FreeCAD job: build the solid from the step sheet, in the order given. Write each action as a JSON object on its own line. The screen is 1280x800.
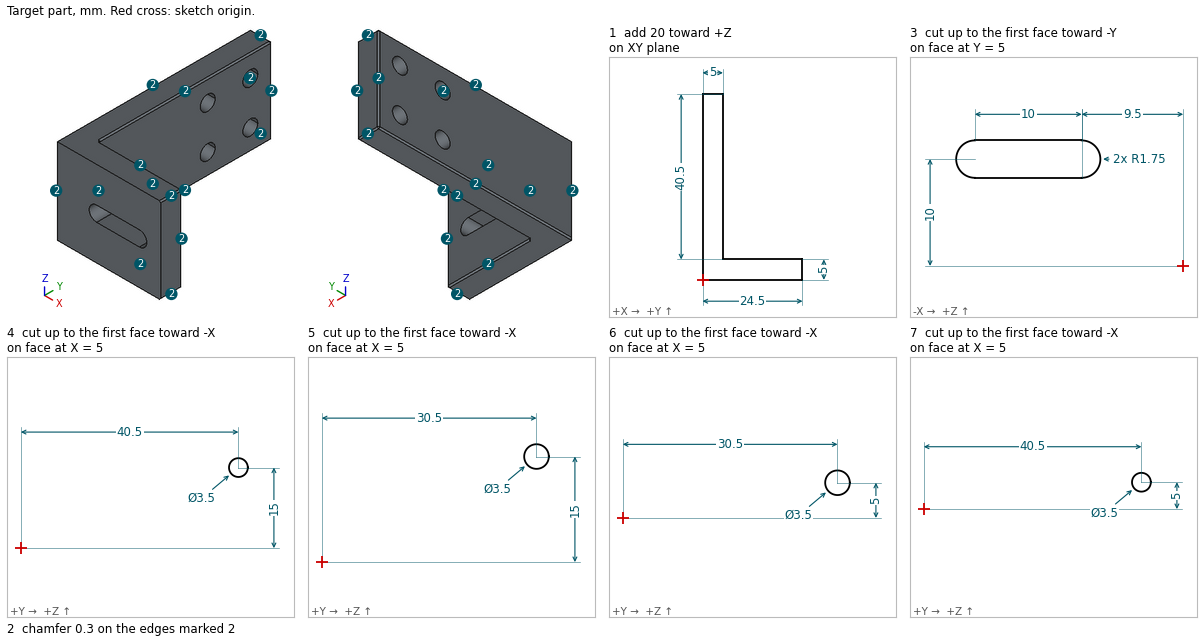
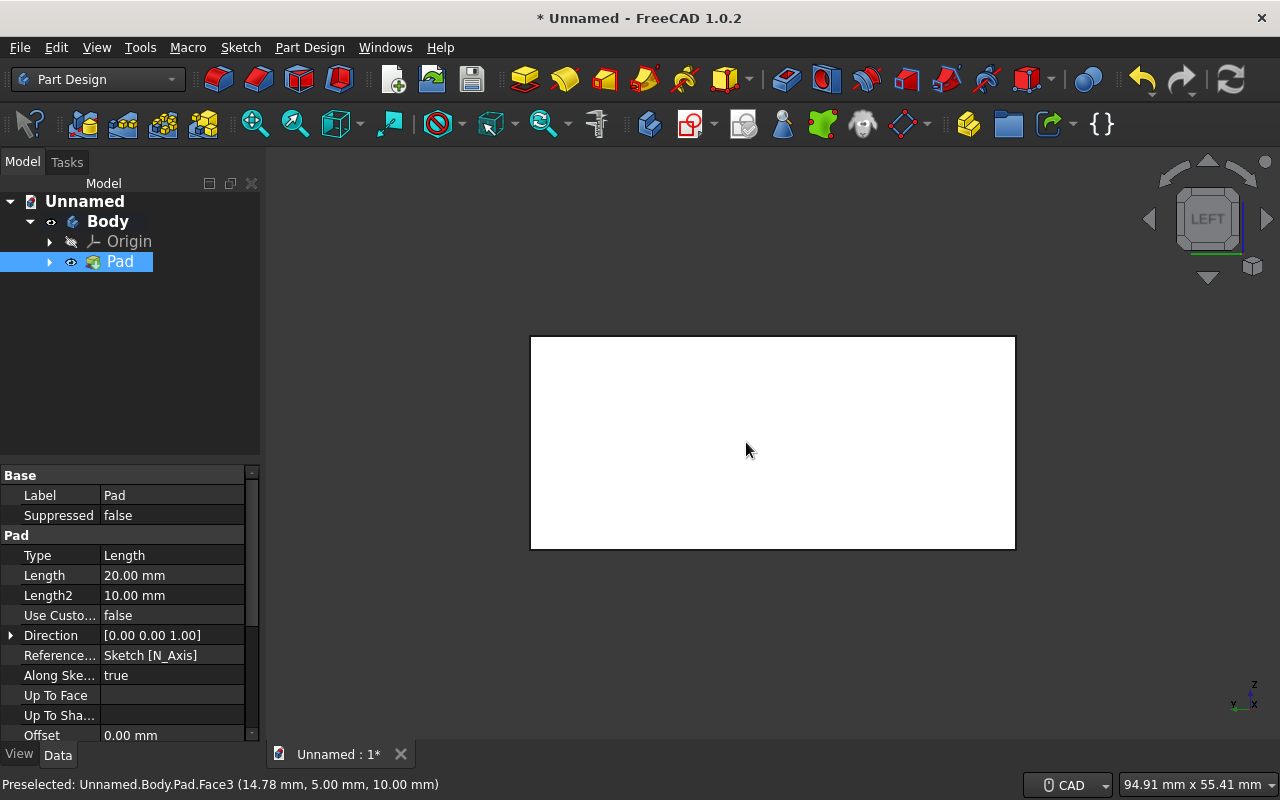
{"action": "left_click", "coordinate": [704, 442], "text": "ctrl"}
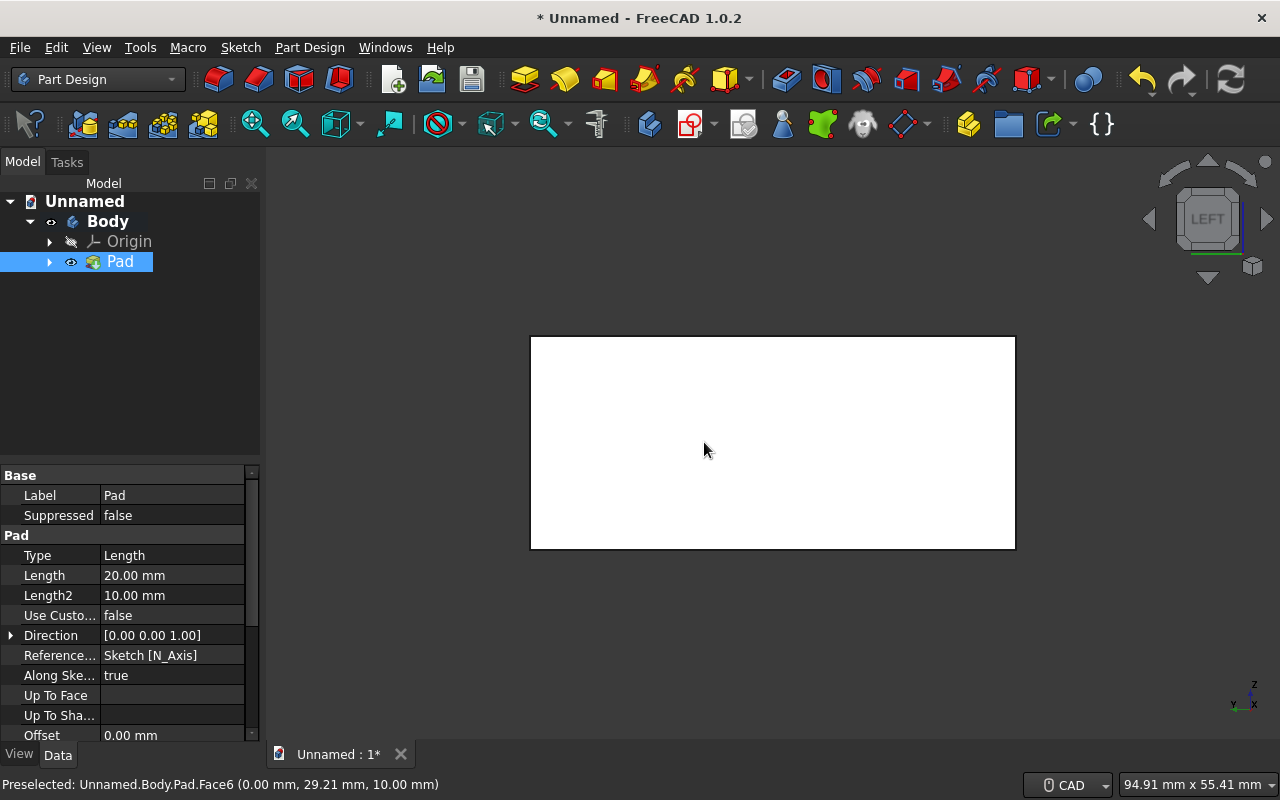
{"action": "left_click", "coordinate": [260, 80]}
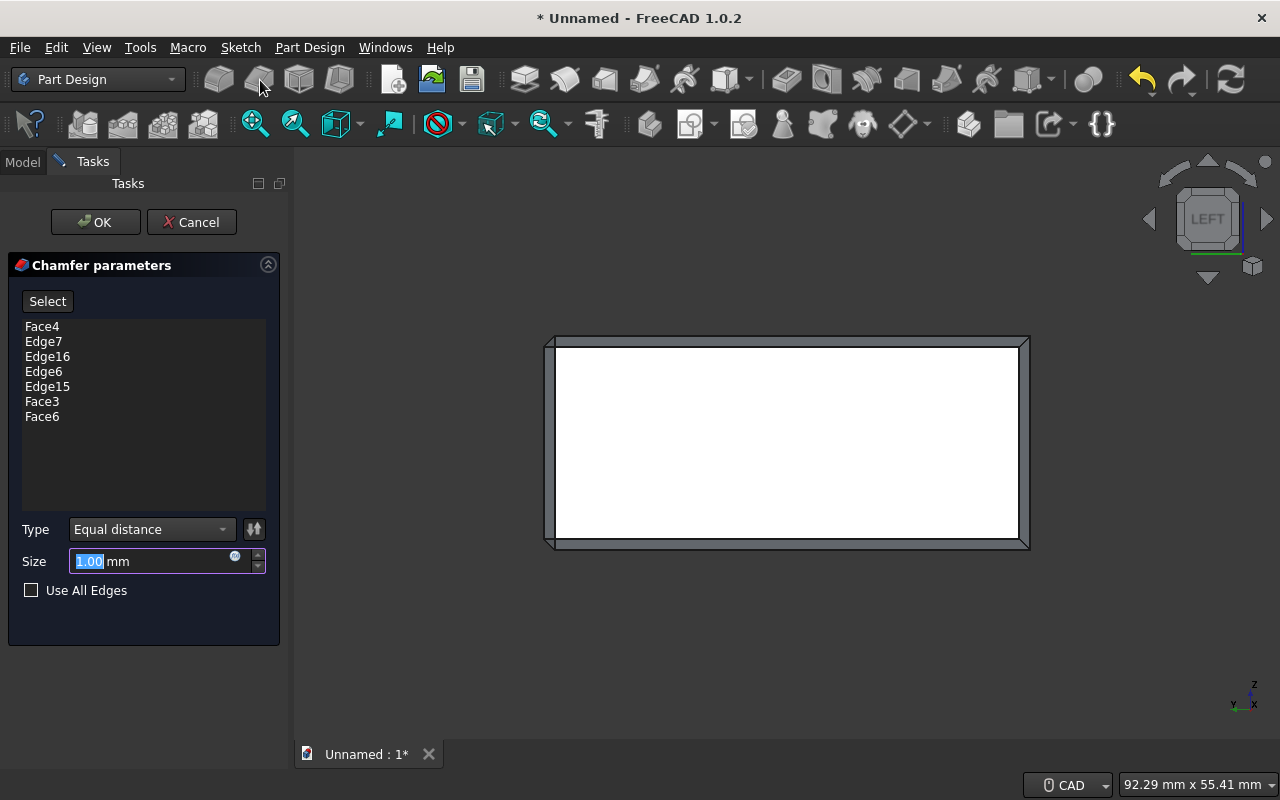
{"action": "type", "text": "0.3"}
{"action": "key", "text": "Tab"}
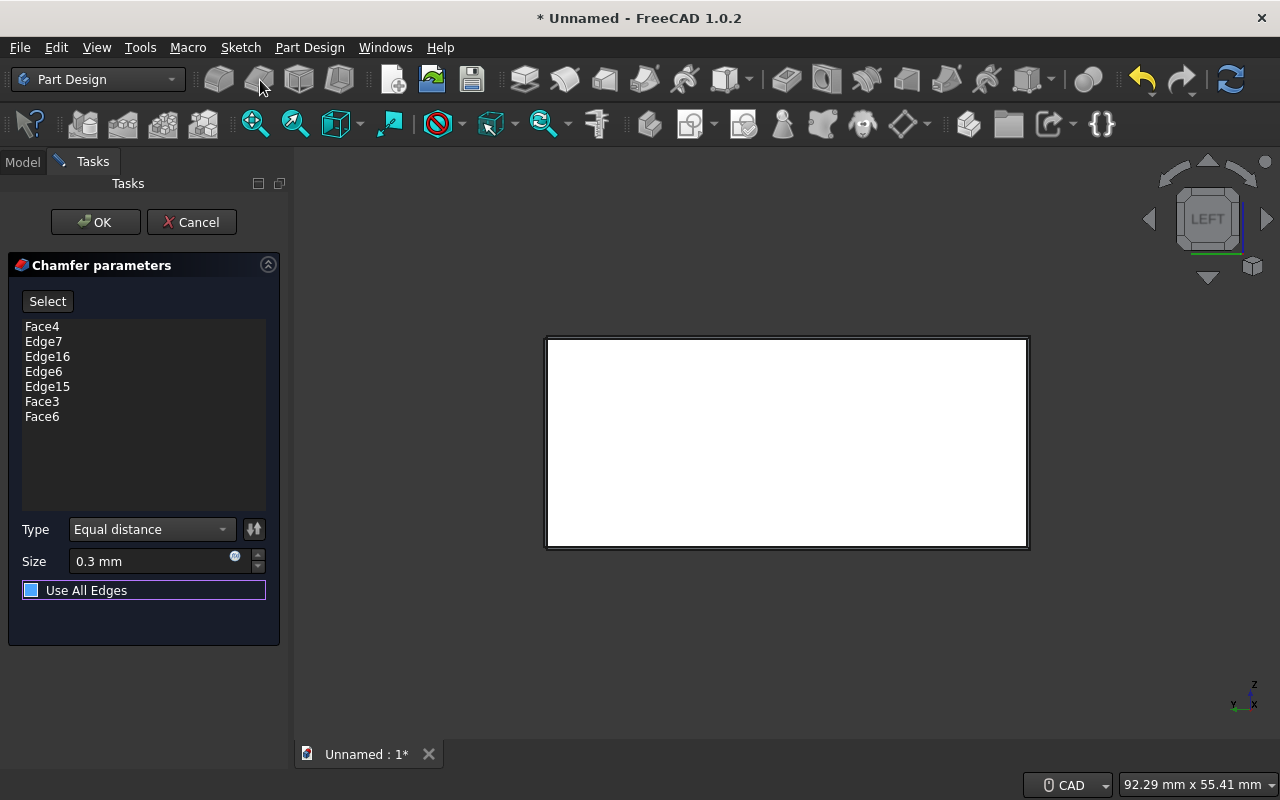
{"action": "left_click", "coordinate": [96, 222]}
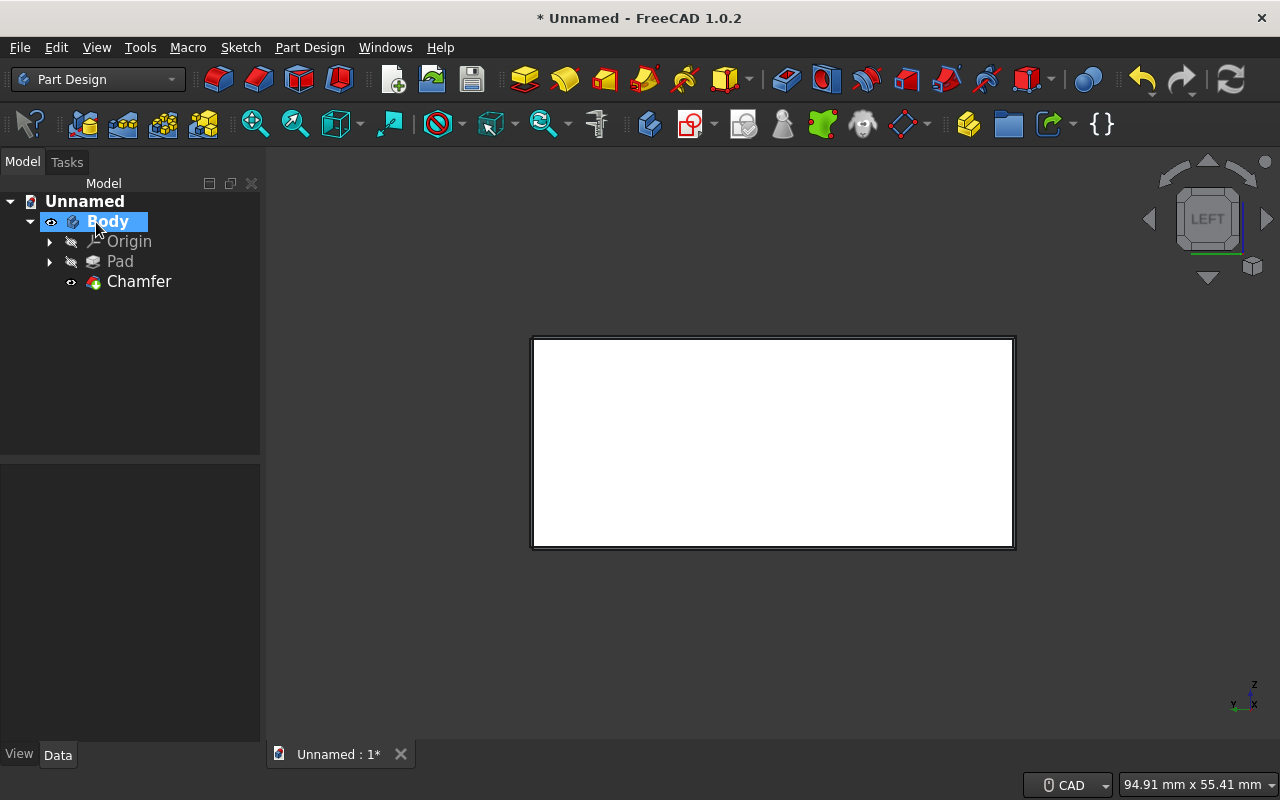
{"action": "key", "text": "4"}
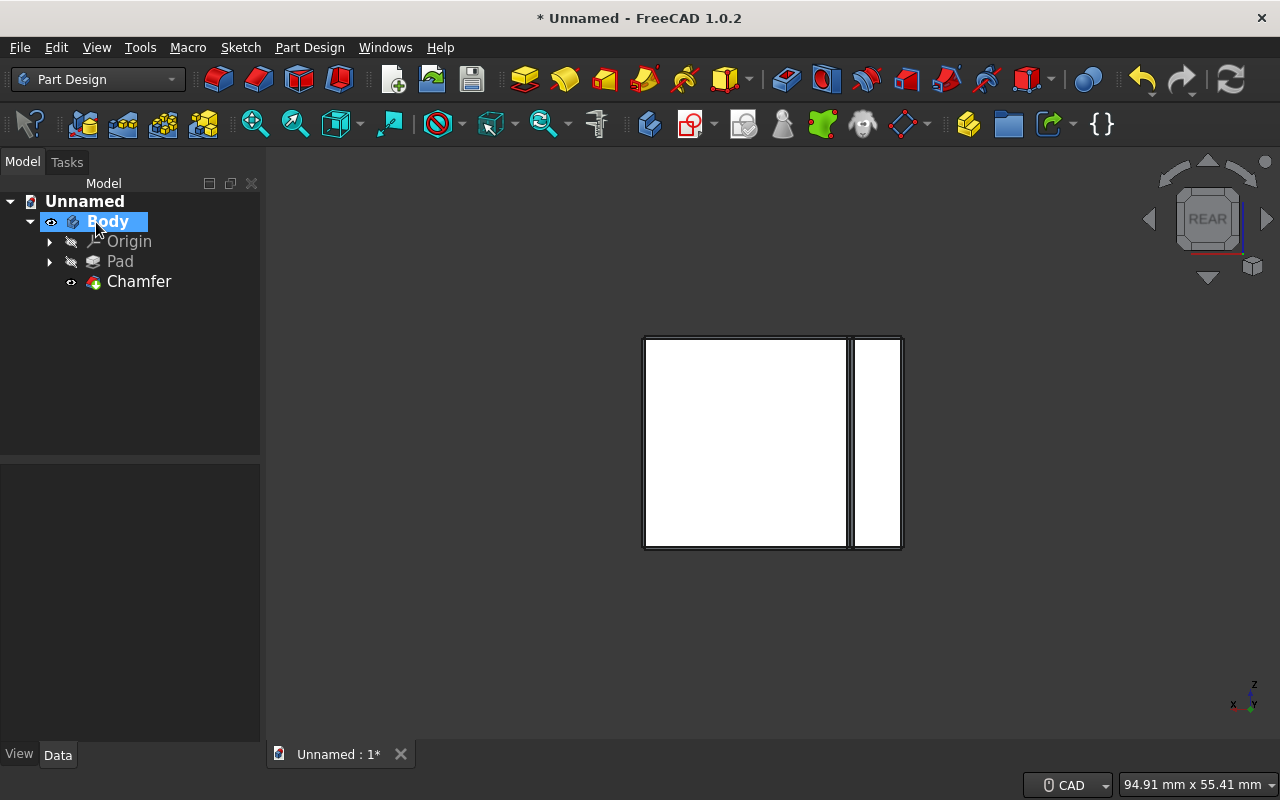
{"action": "left_click", "coordinate": [256, 124]}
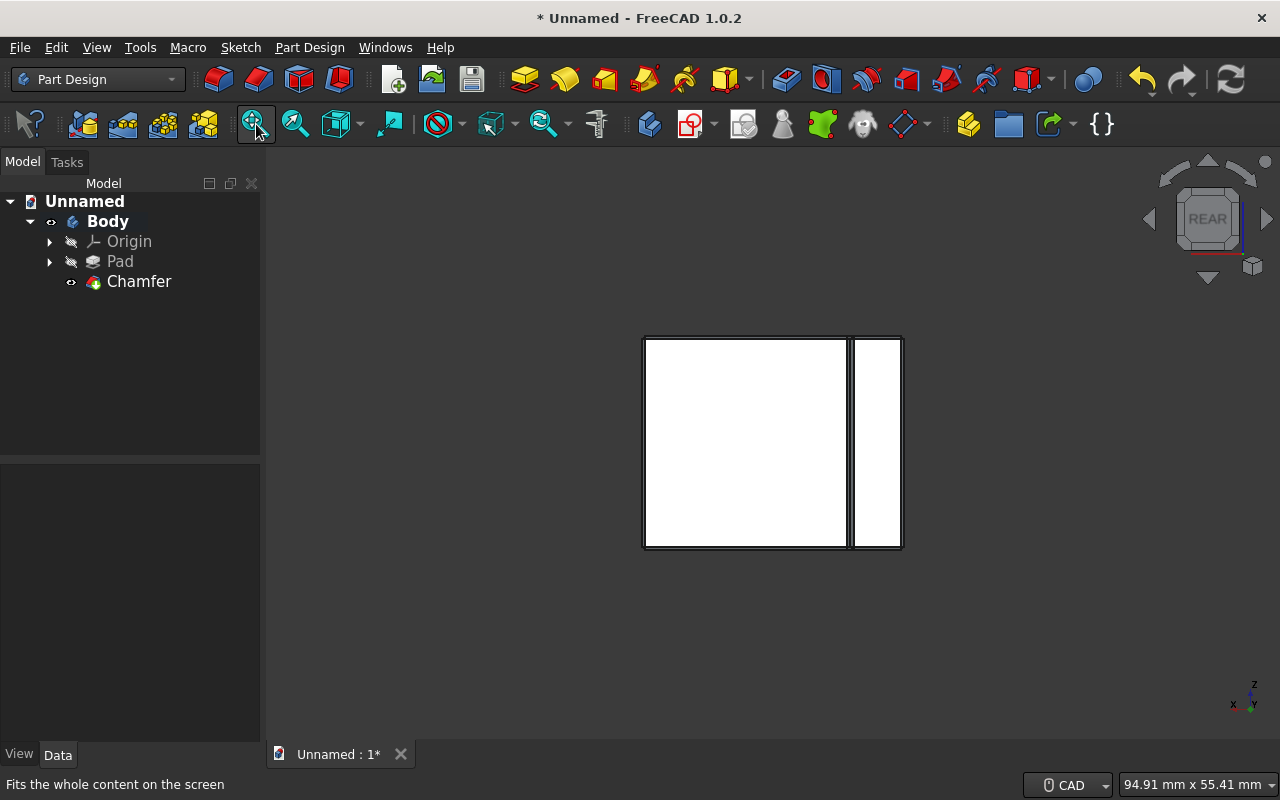
{"action": "left_click", "coordinate": [746, 442]}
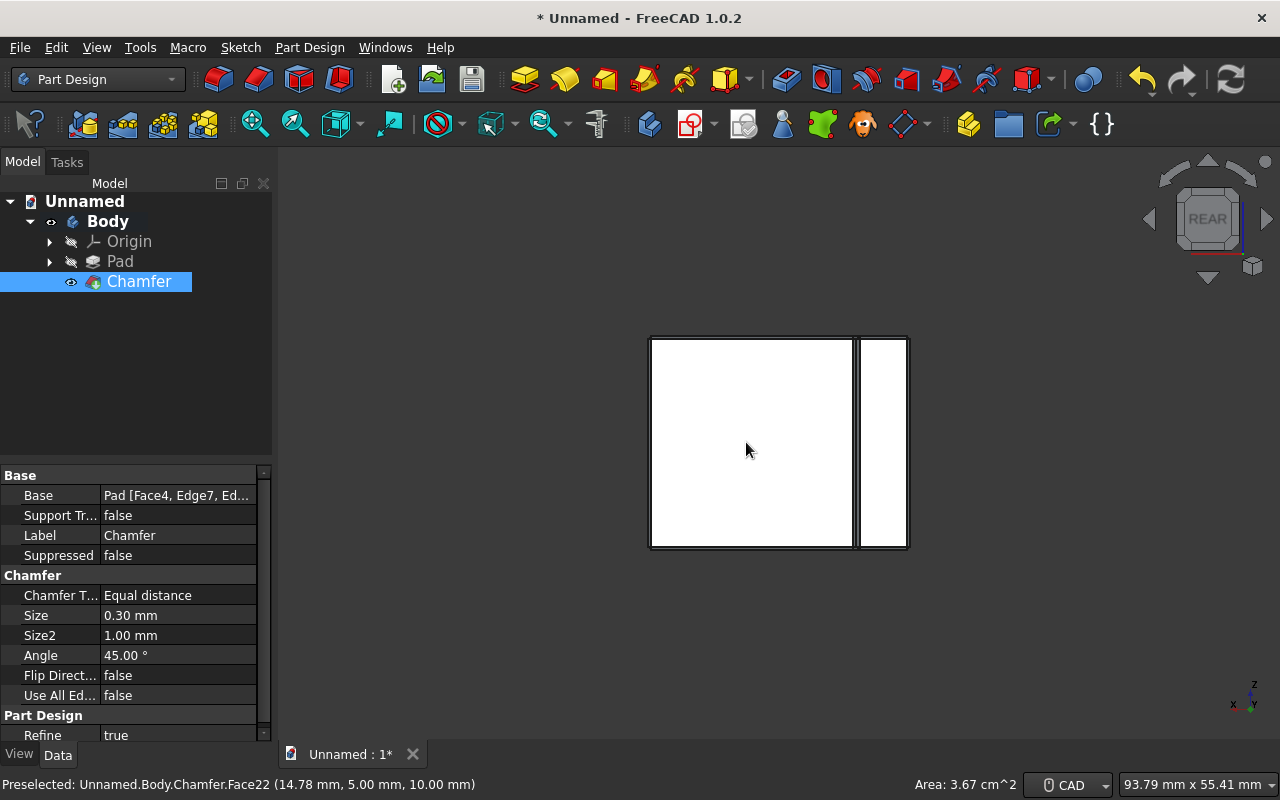
{"action": "left_click", "coordinate": [690, 124]}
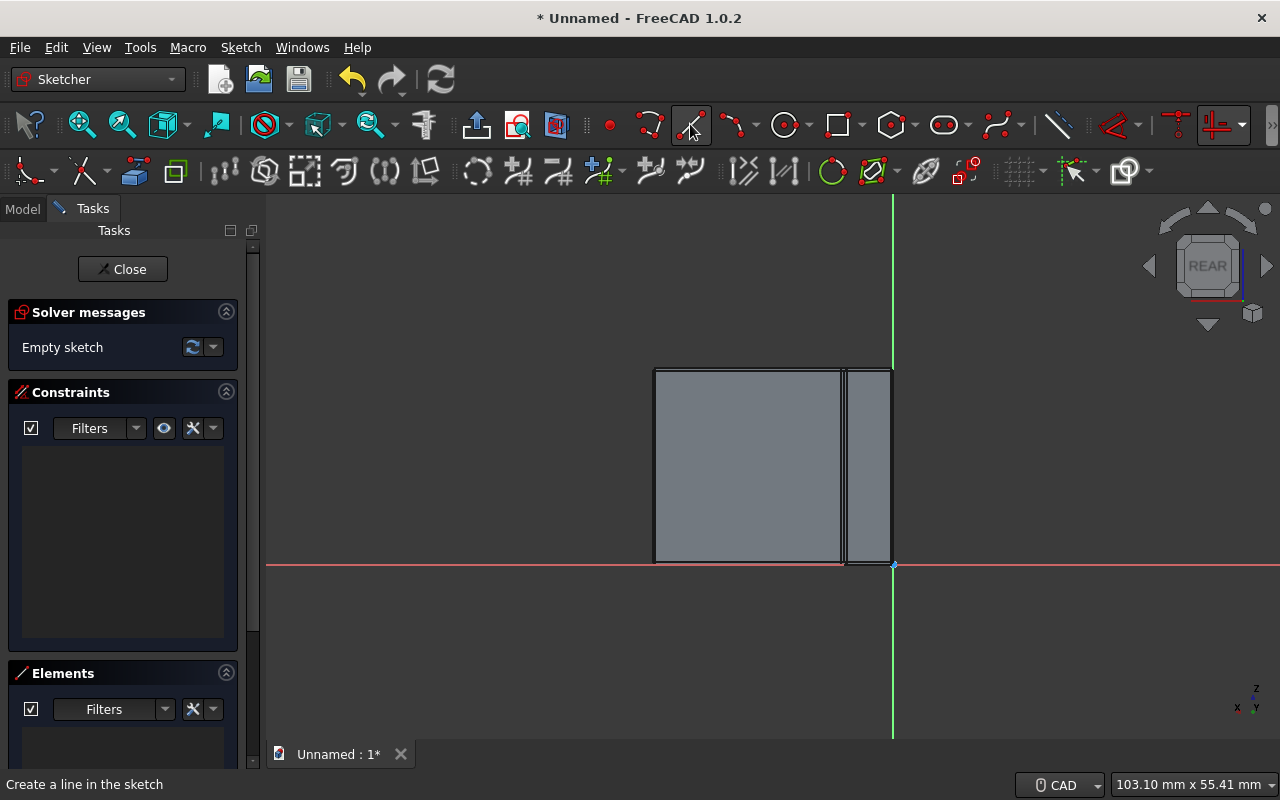
{"action": "scroll", "coordinate": [838, 531], "scroll_direction": "up", "scroll_amount": 5}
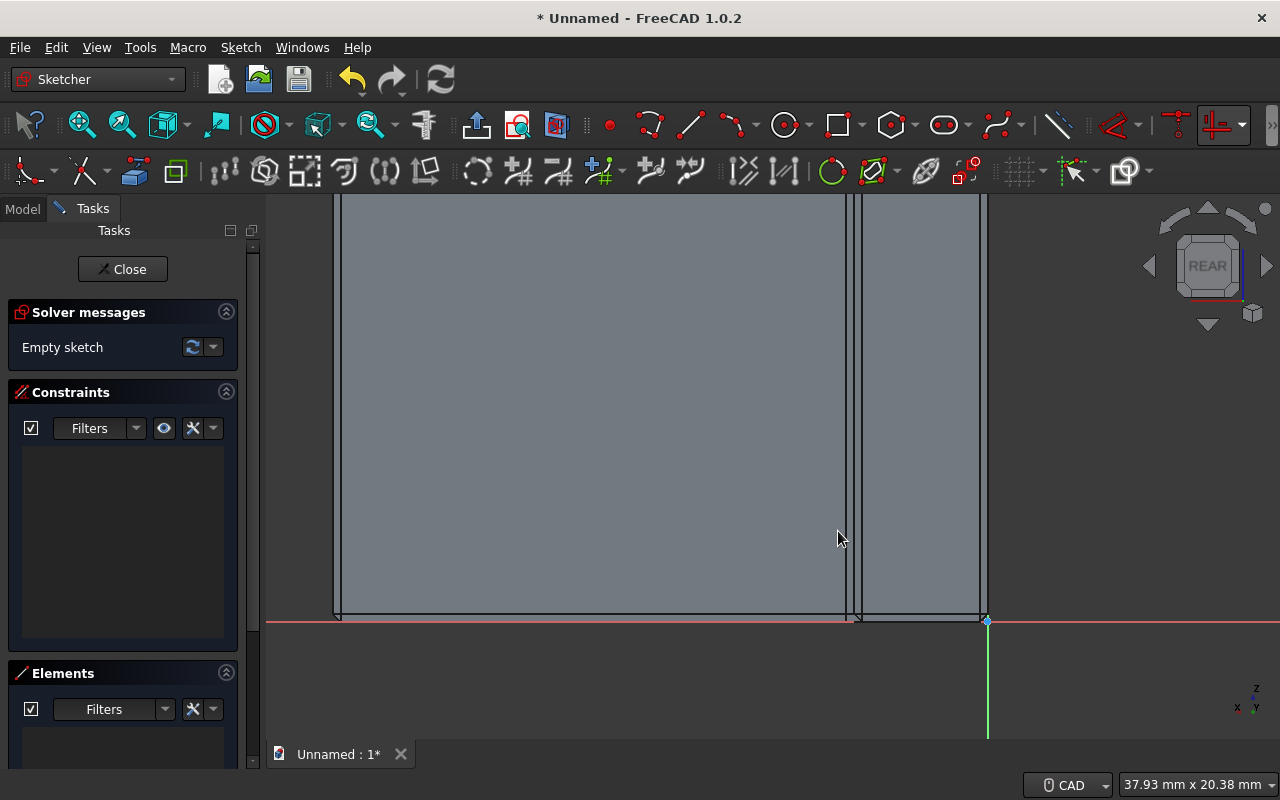
{"action": "key", "text": "g s"}